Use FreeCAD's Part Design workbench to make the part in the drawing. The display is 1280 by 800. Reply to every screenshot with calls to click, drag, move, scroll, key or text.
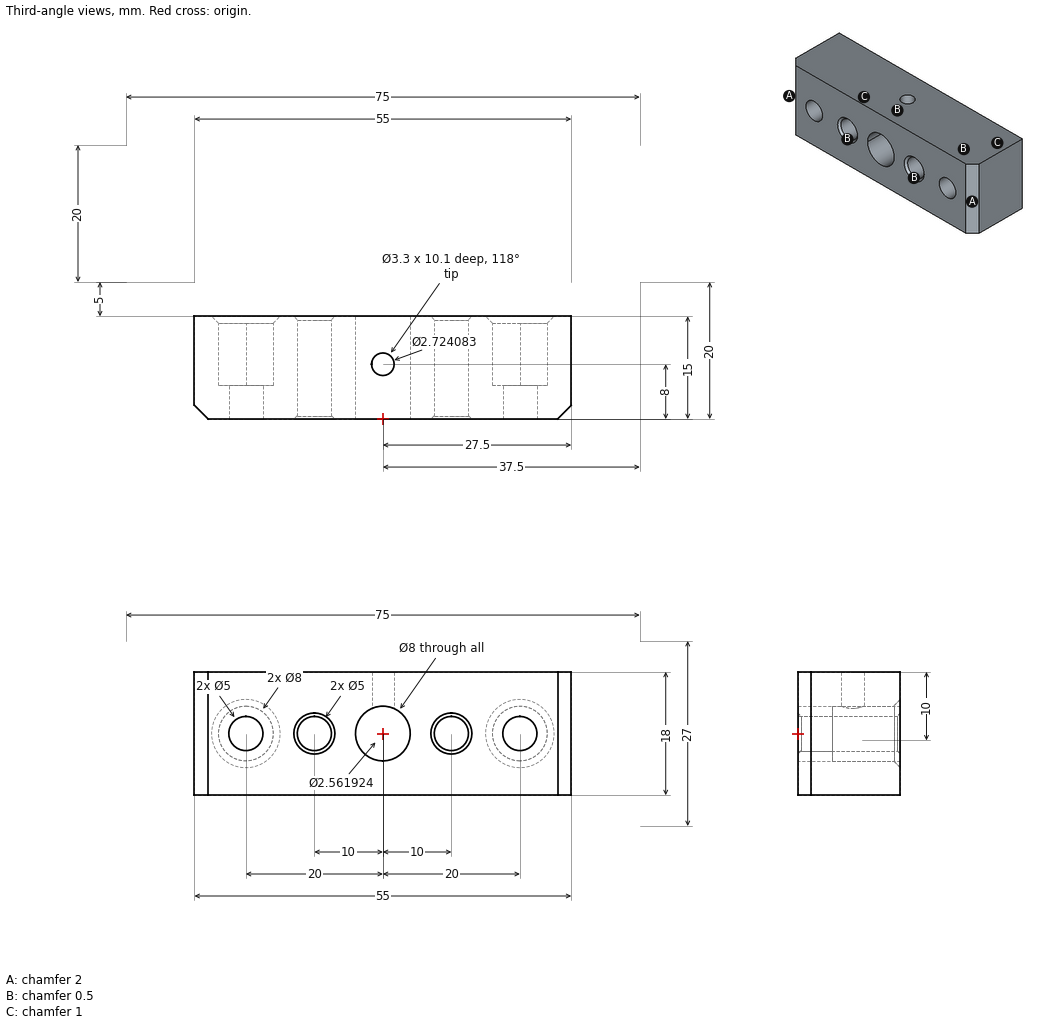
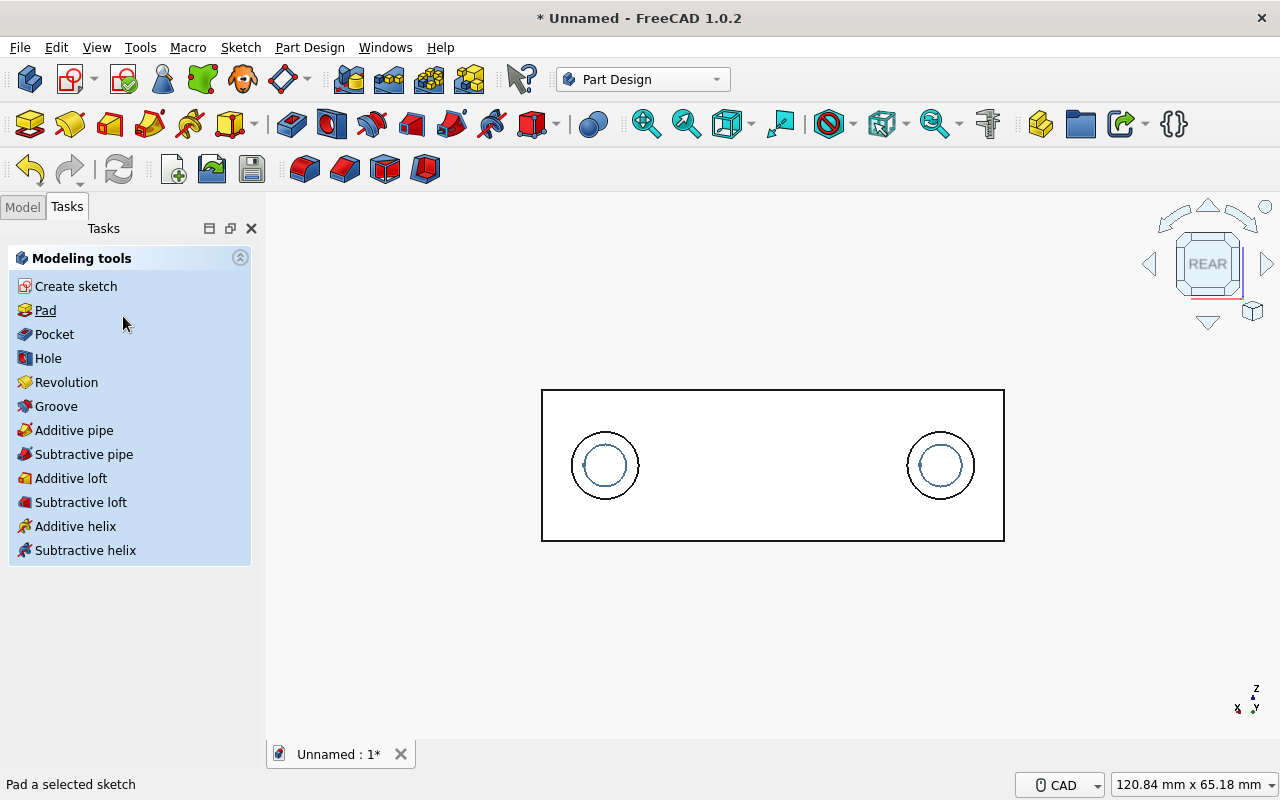
click(292, 124)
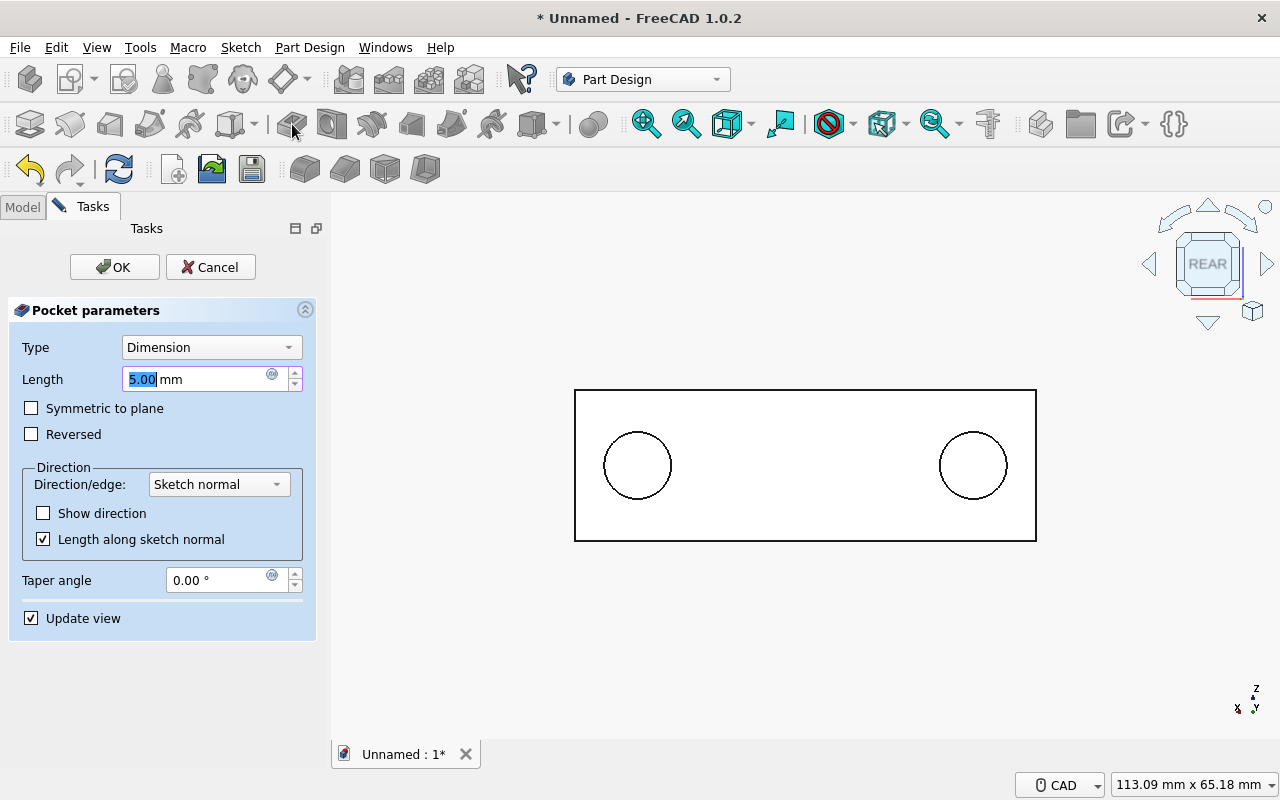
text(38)
key(Tab)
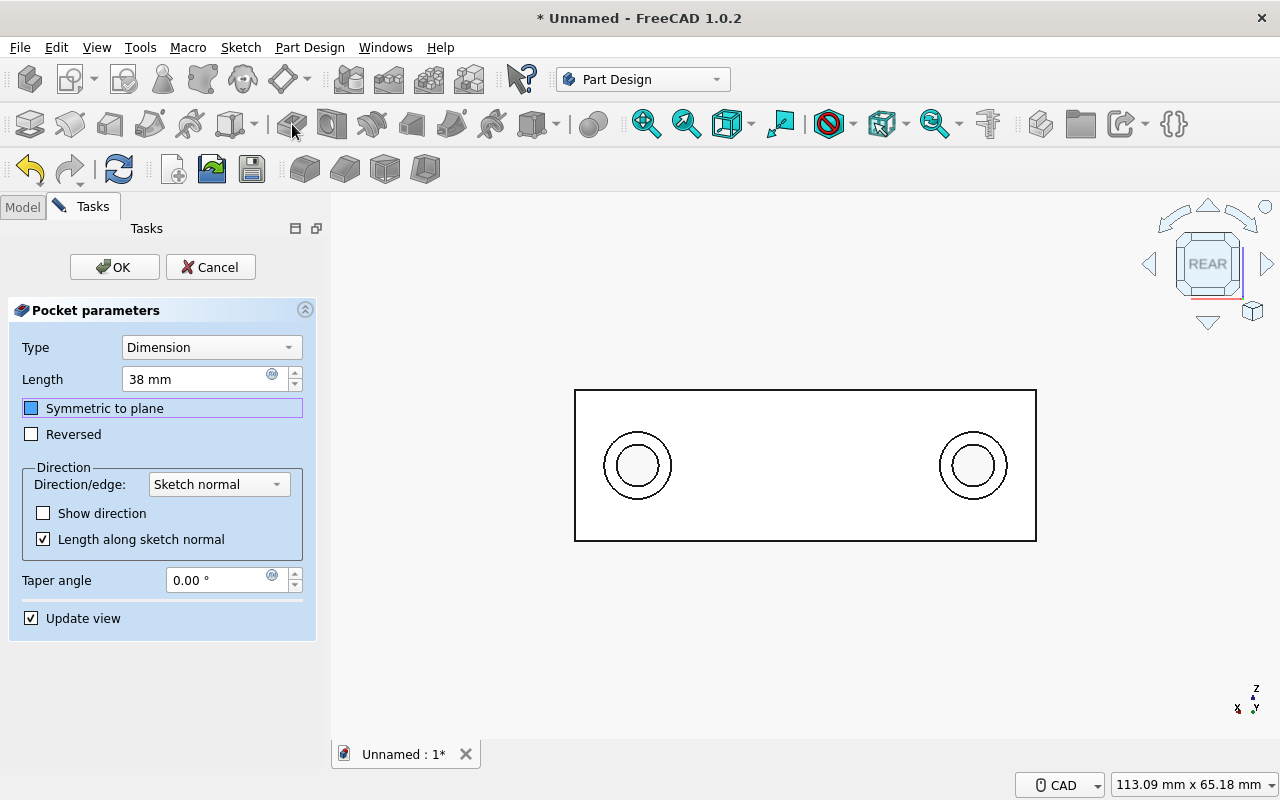
click(115, 267)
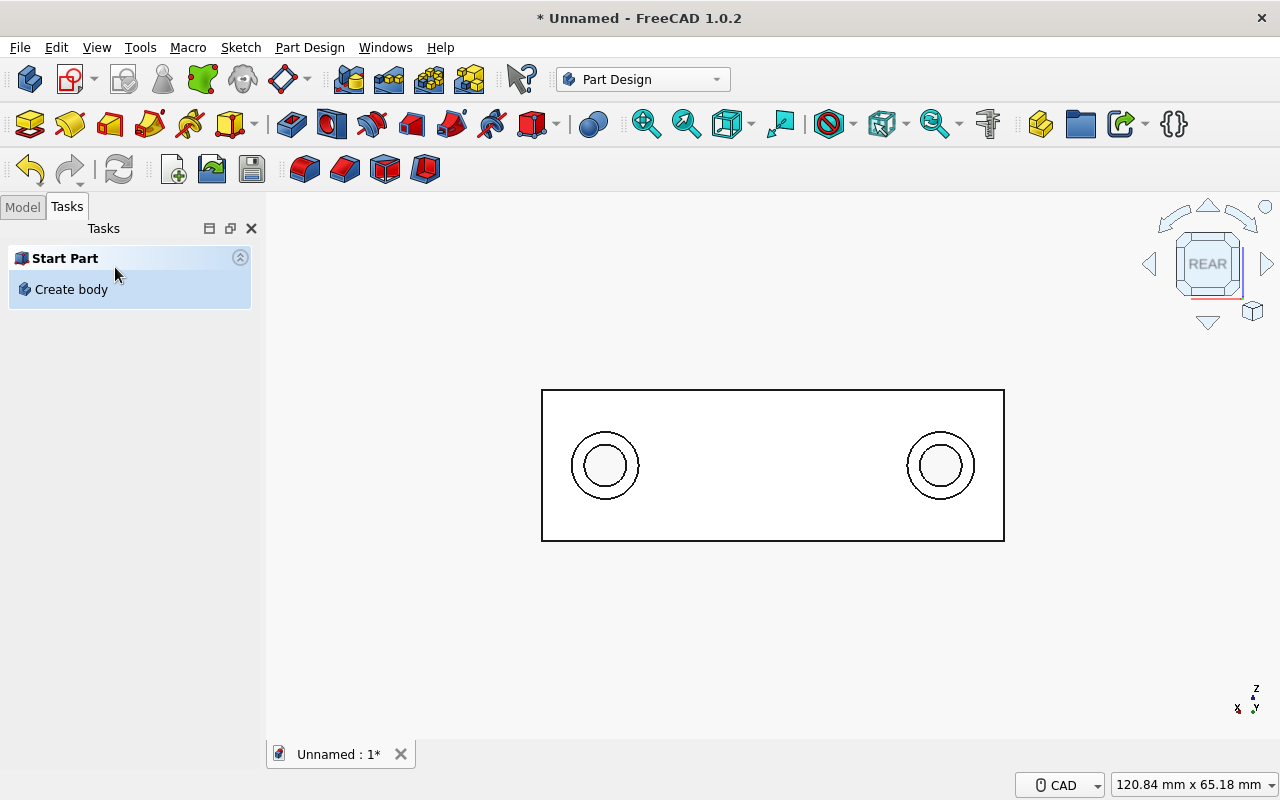
click(773, 465)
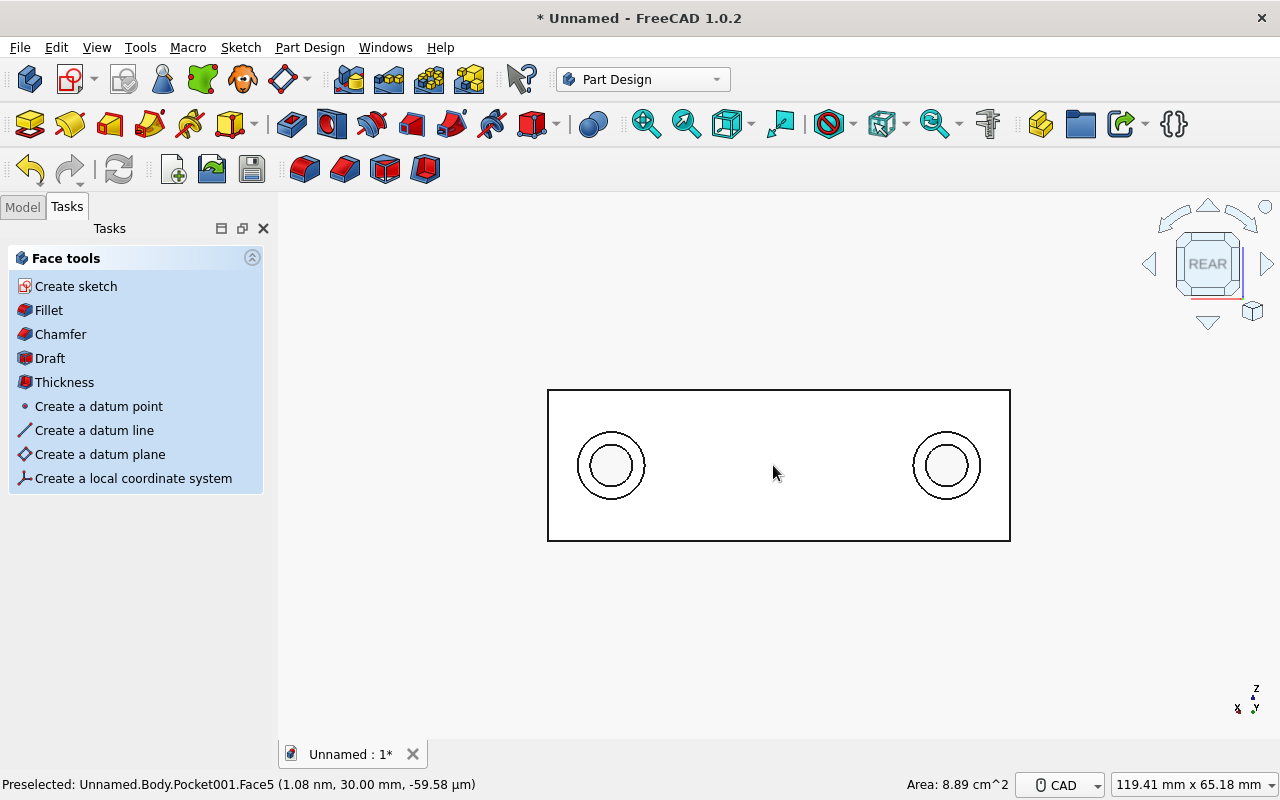
click(70, 80)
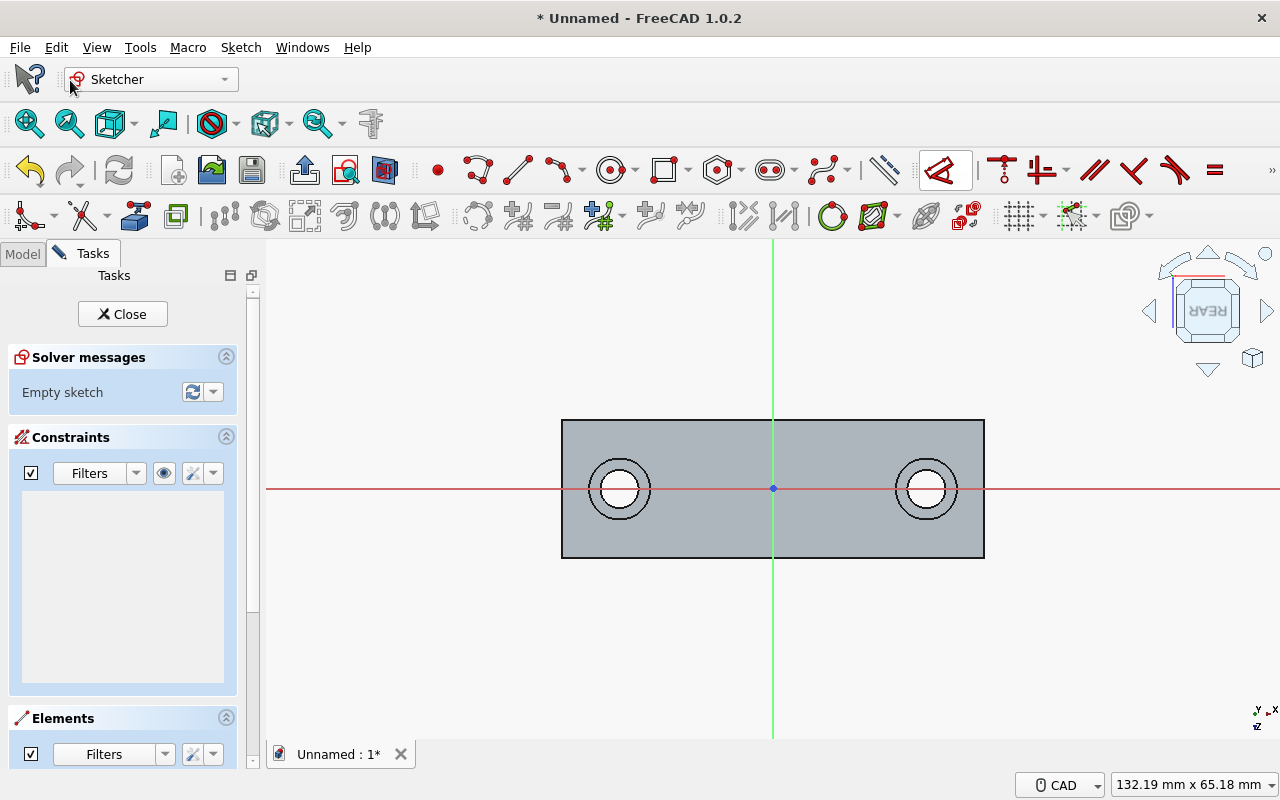
key(g)
key(v)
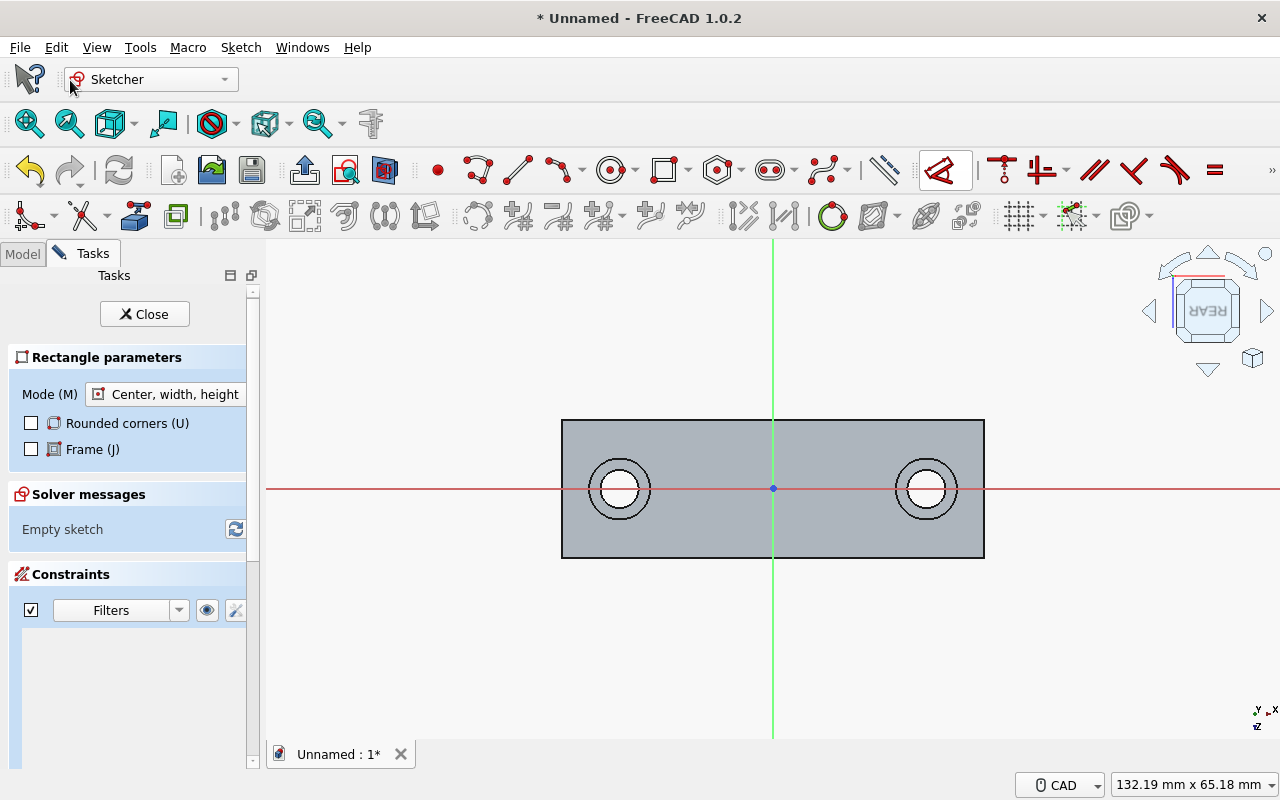
click(773, 489)
move(1061, 385)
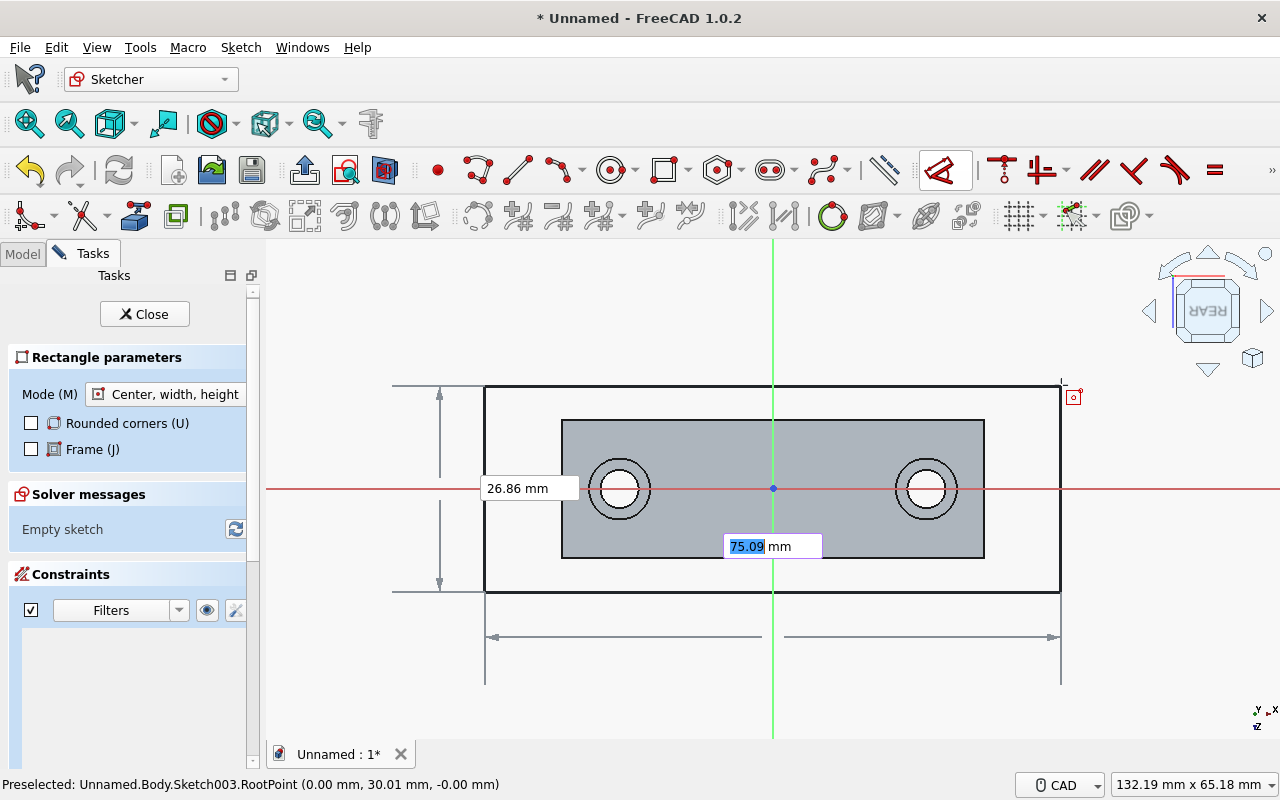
text(75)
key(Tab)
text(27)
key(Return)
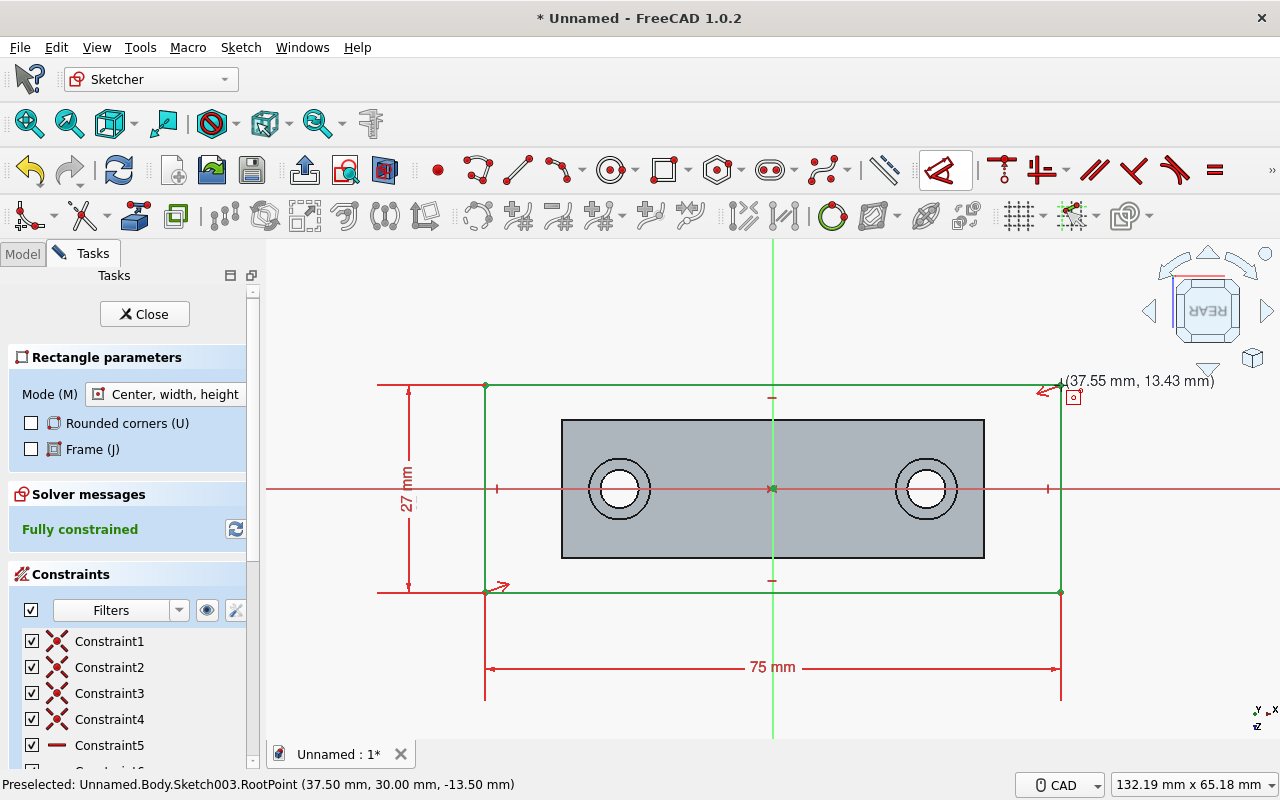
click(612, 170)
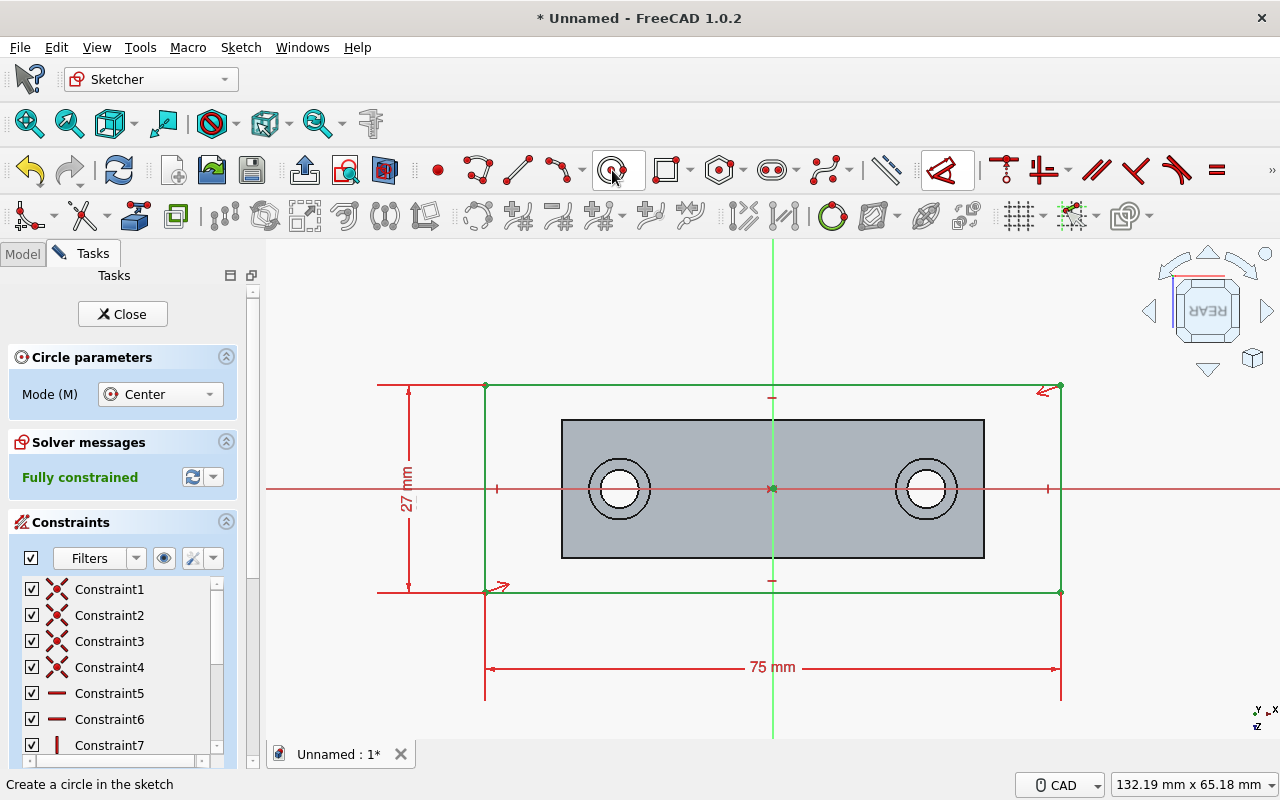
click(620, 489)
move(641, 467)